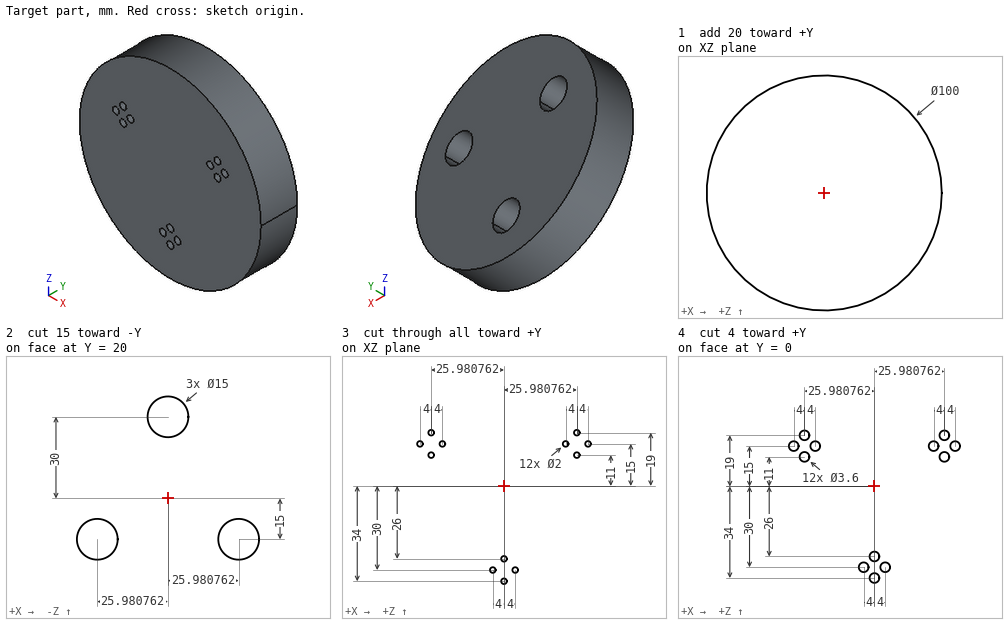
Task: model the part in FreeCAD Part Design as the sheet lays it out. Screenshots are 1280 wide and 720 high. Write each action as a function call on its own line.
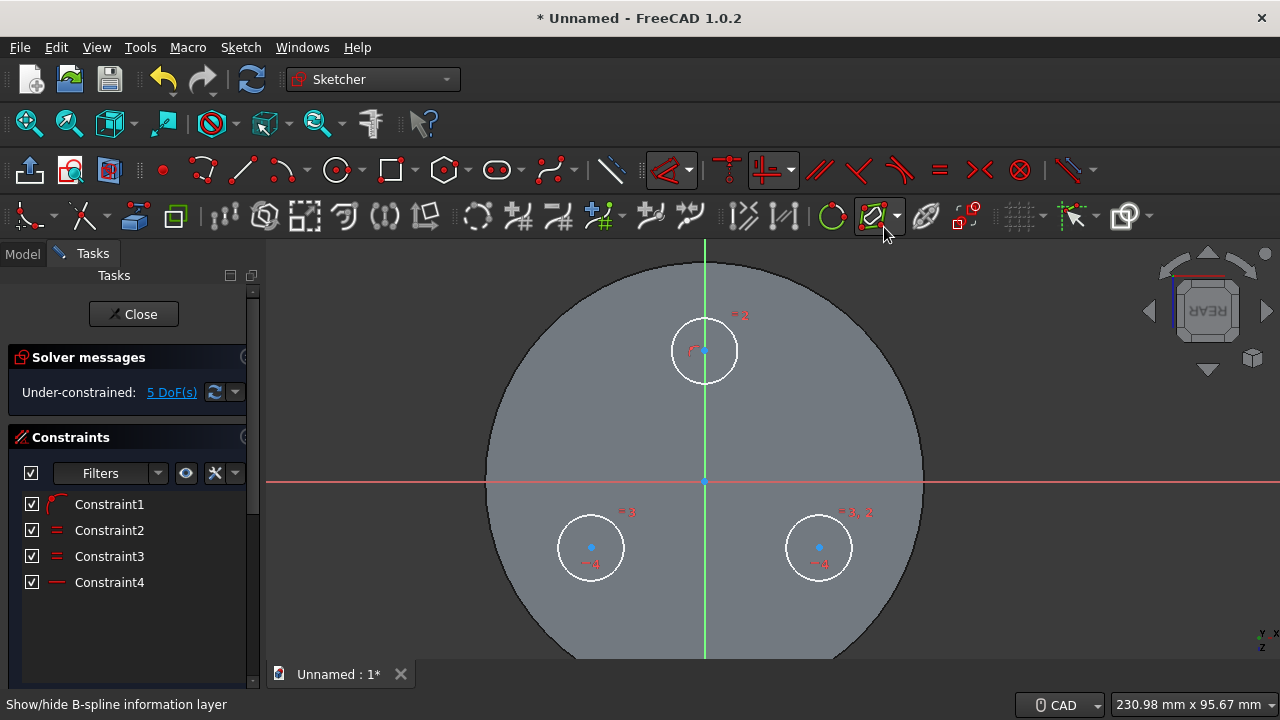
click(728, 328)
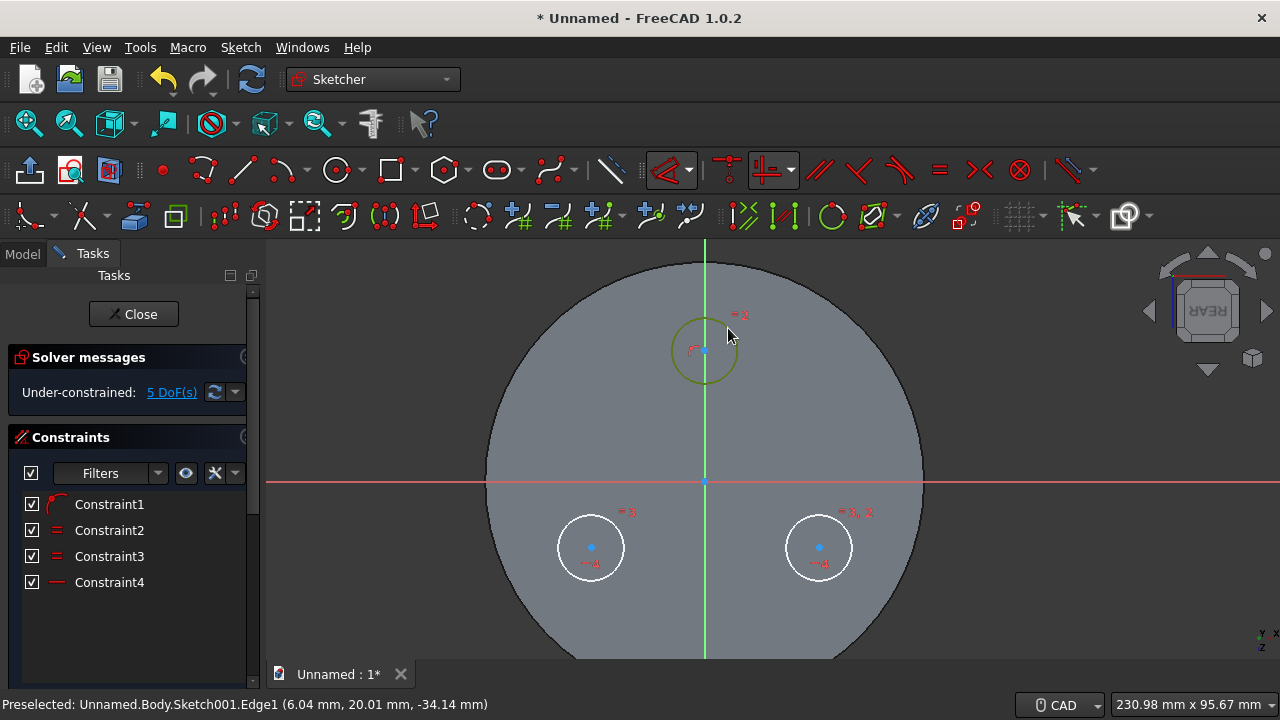
key(k)
key(o)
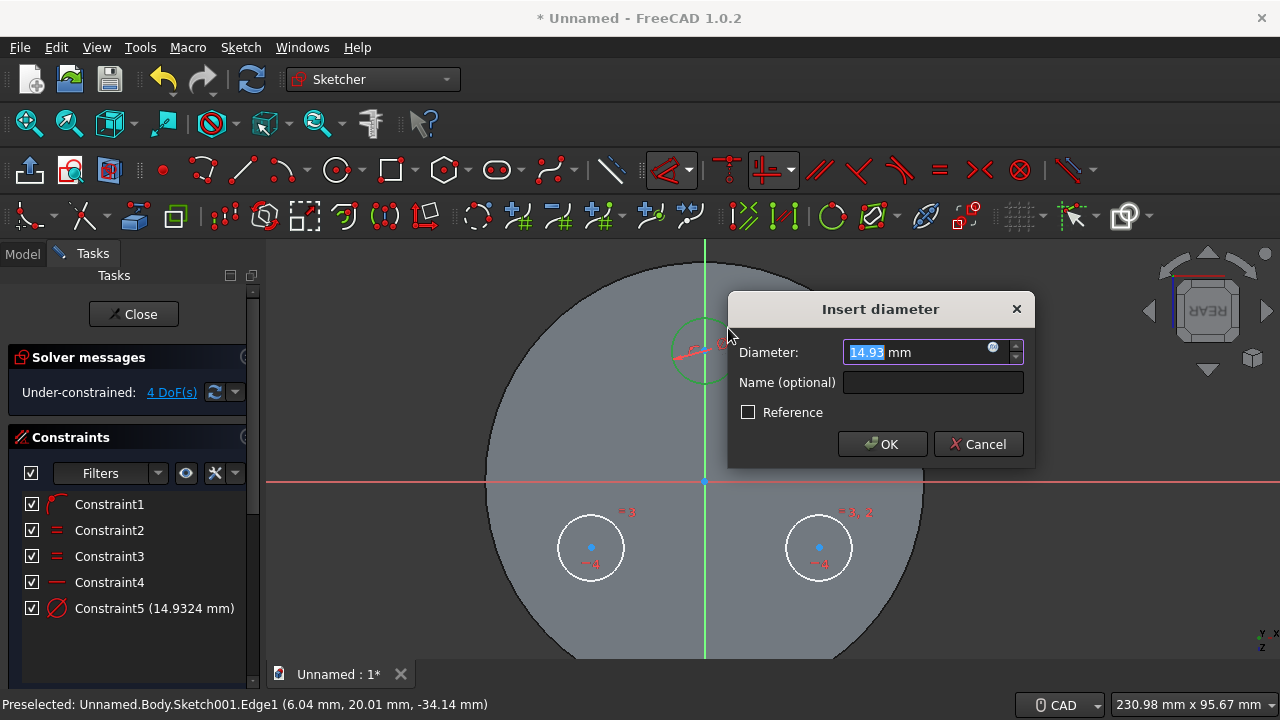
text(15)
key(Return)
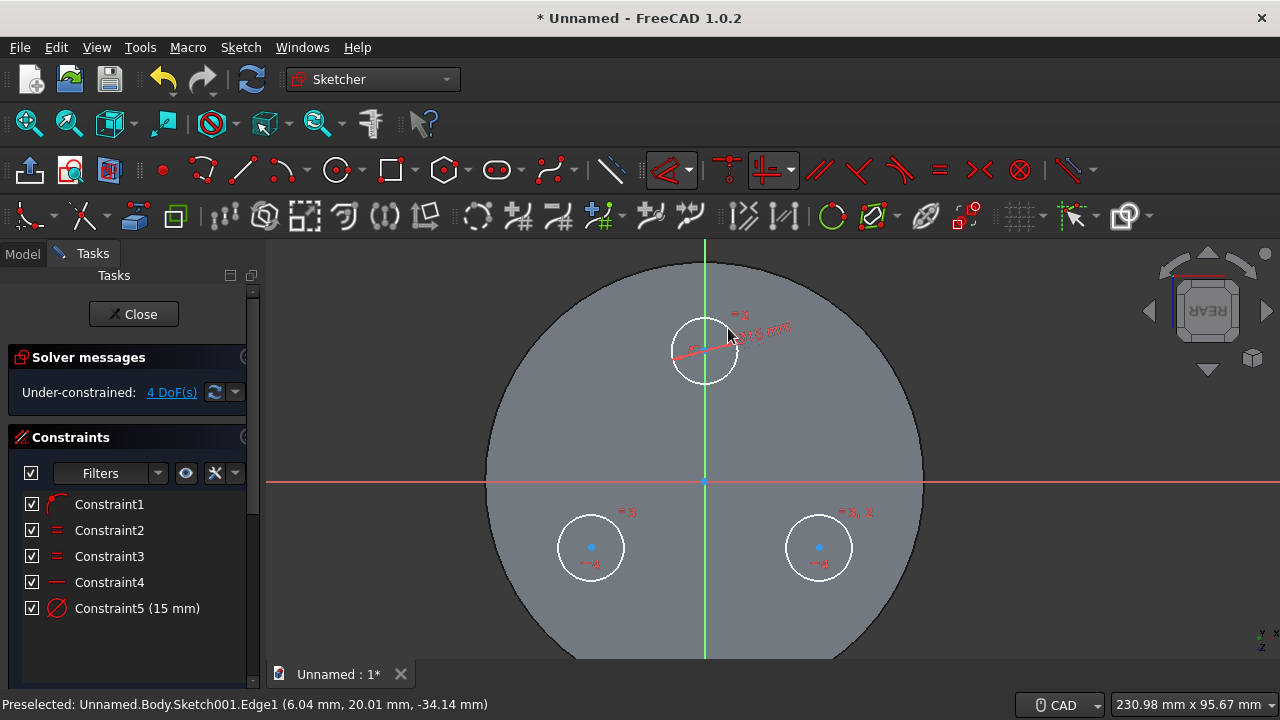
click(705, 351)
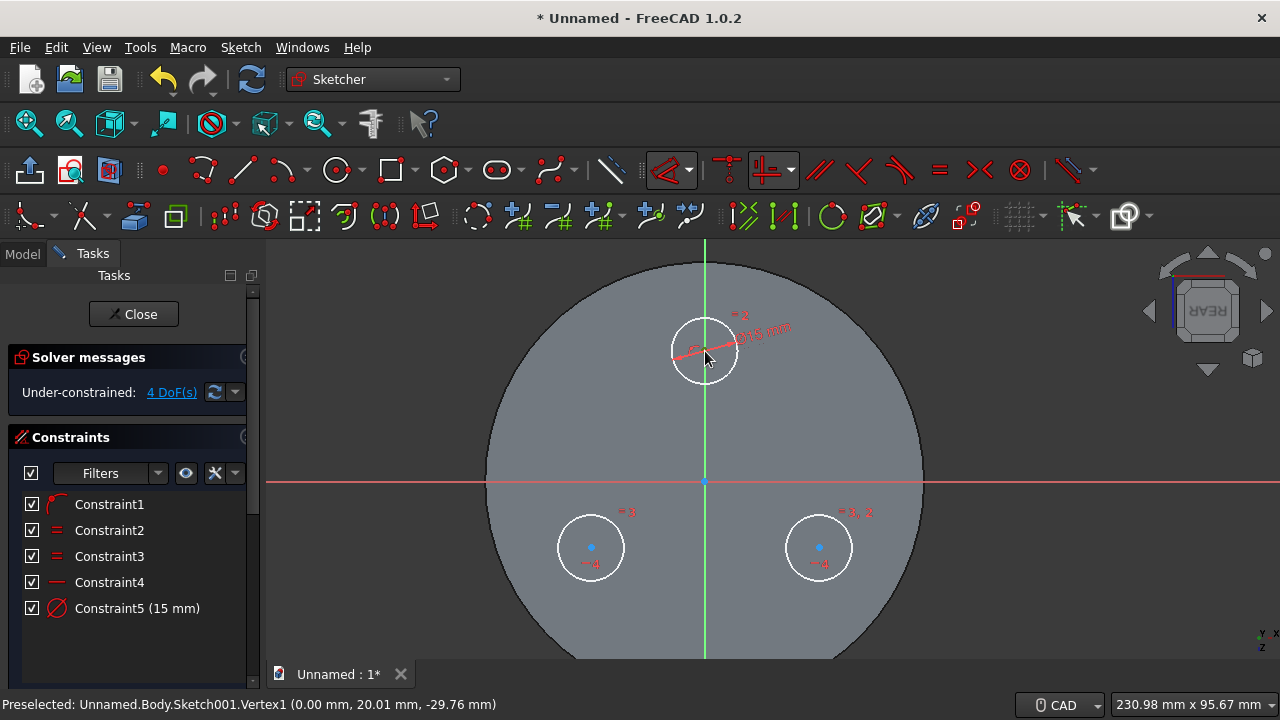
key(i)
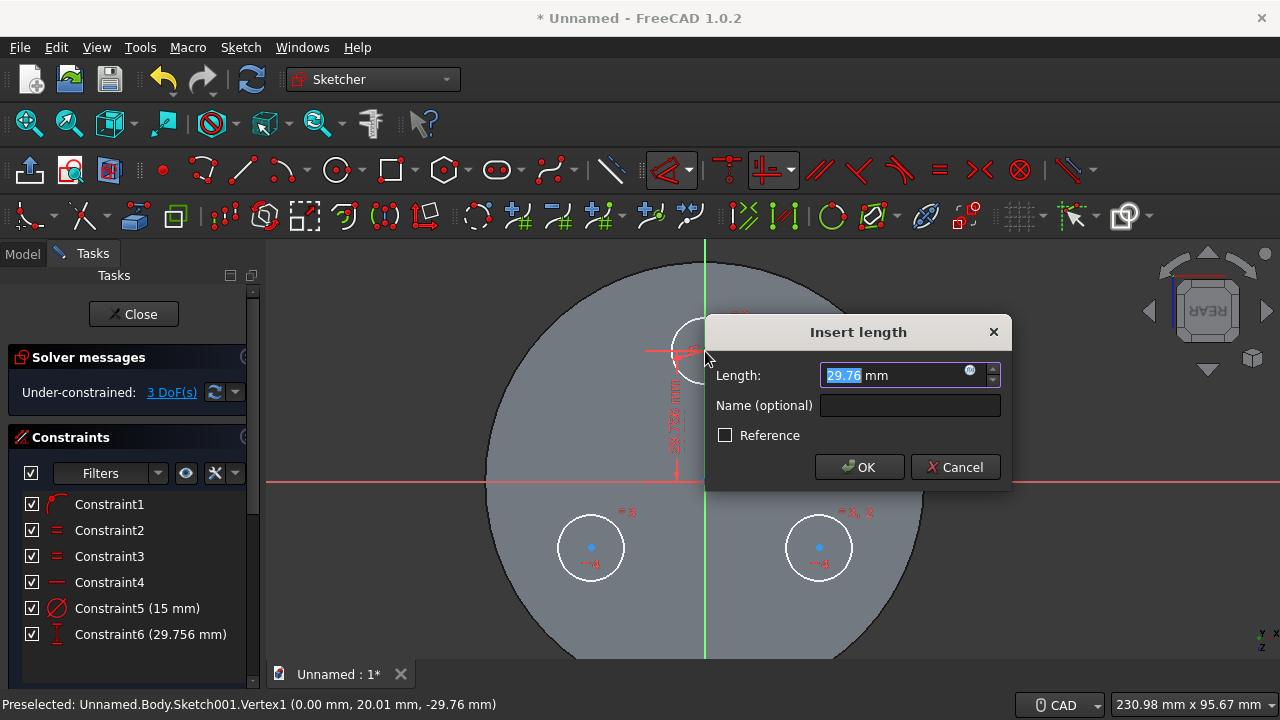
text(30)
key(Return)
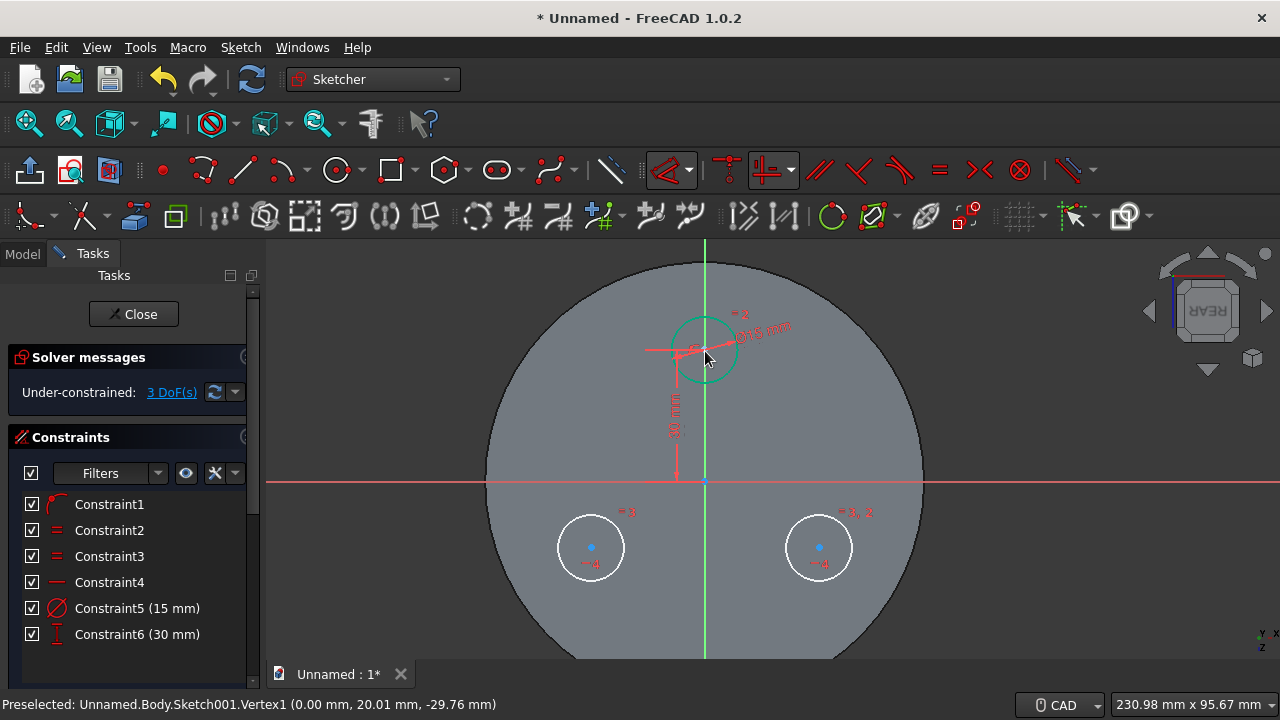
click(819, 548)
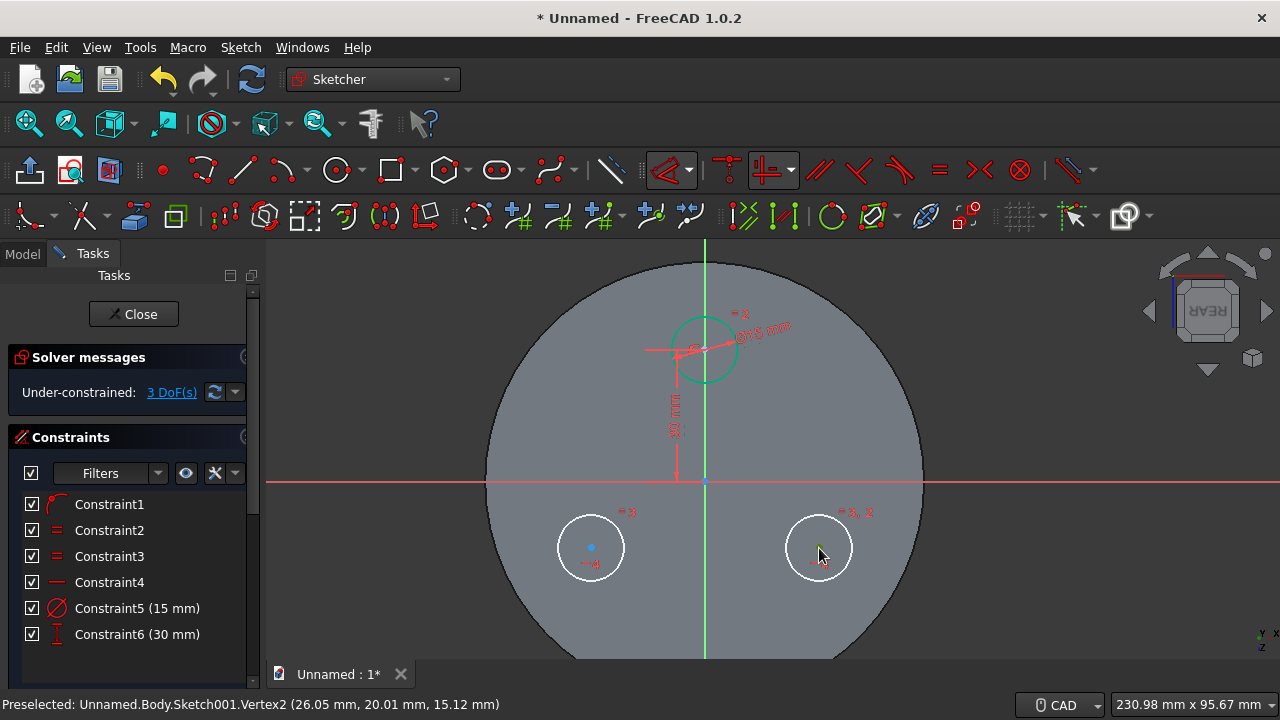
key(i)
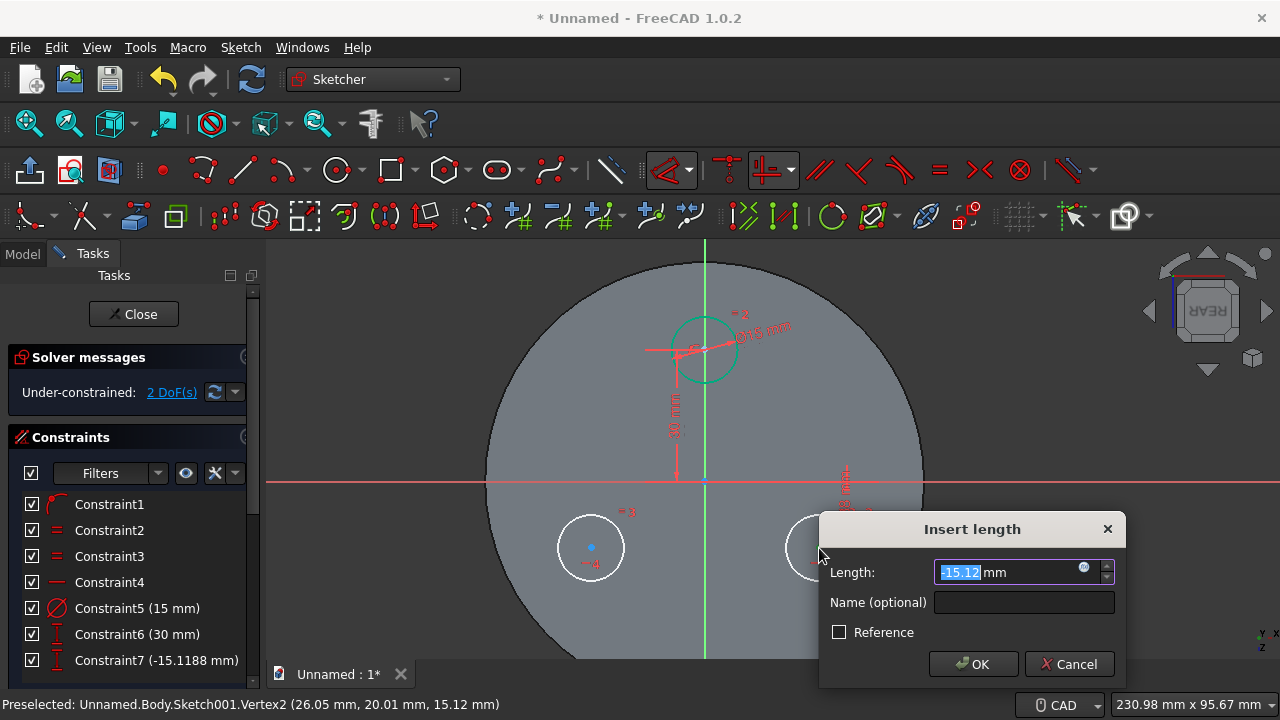
text(-15)
key(Return)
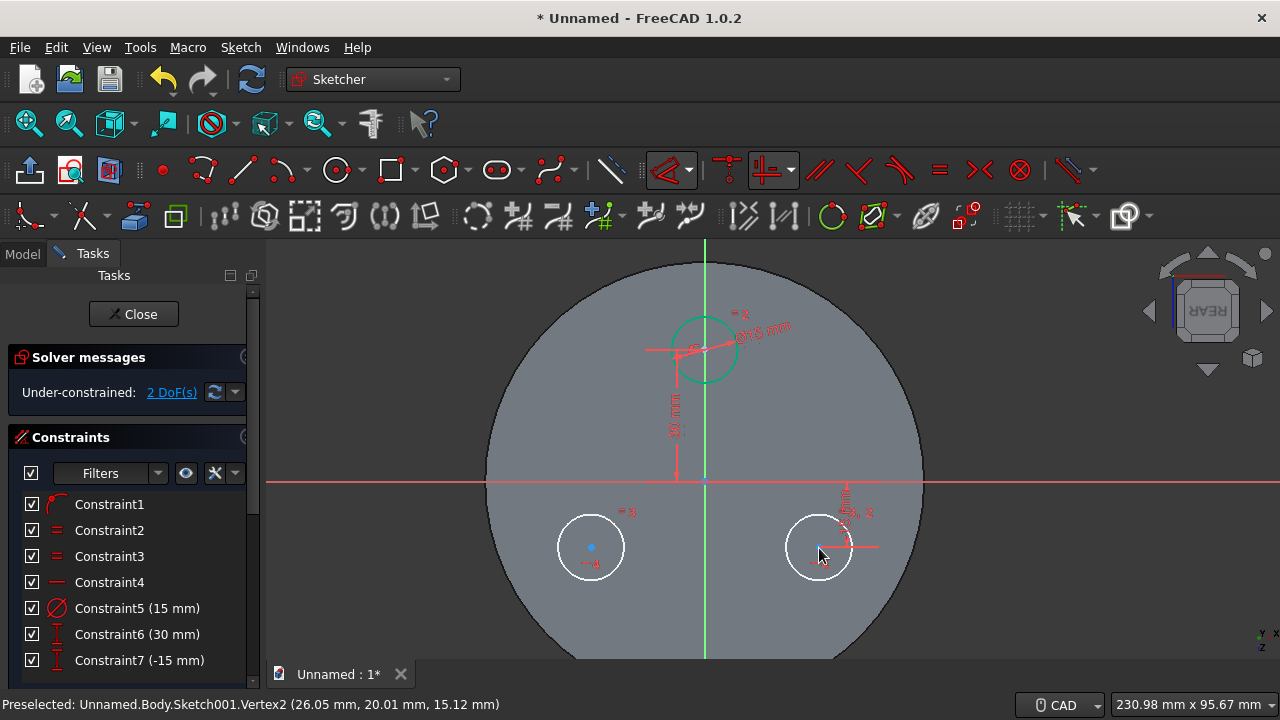
click(819, 547)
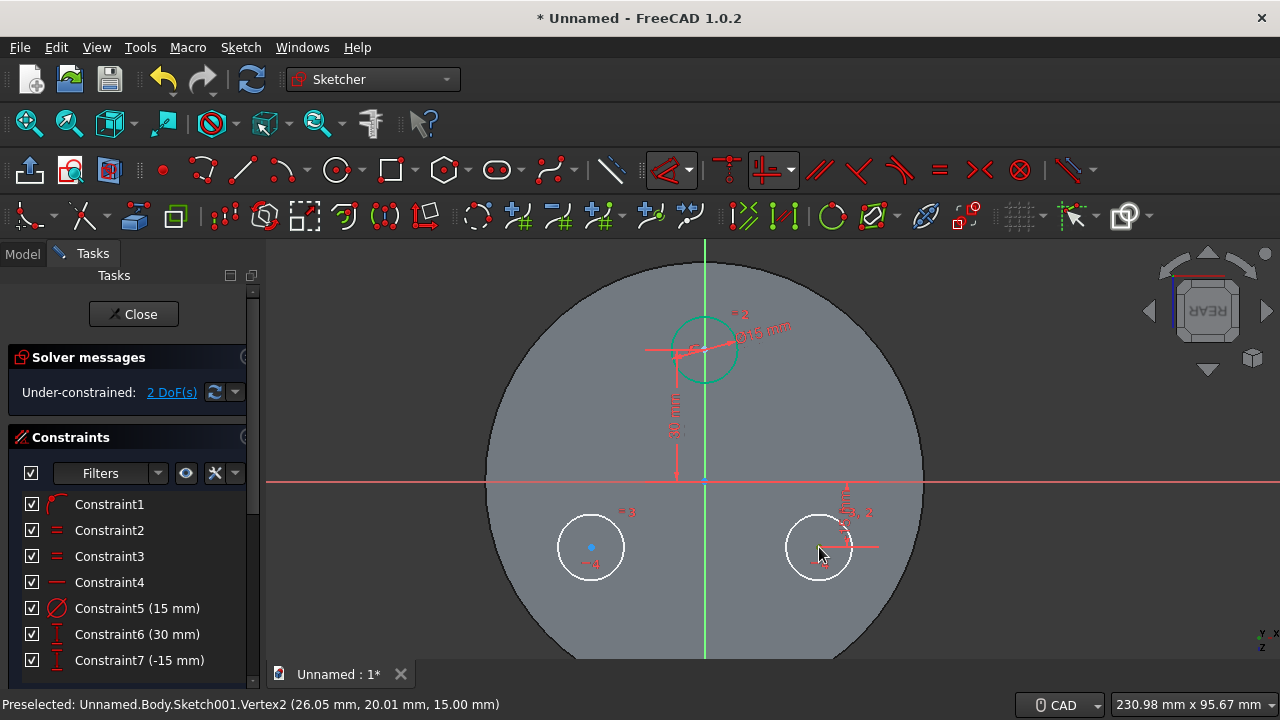
click(692, 170)